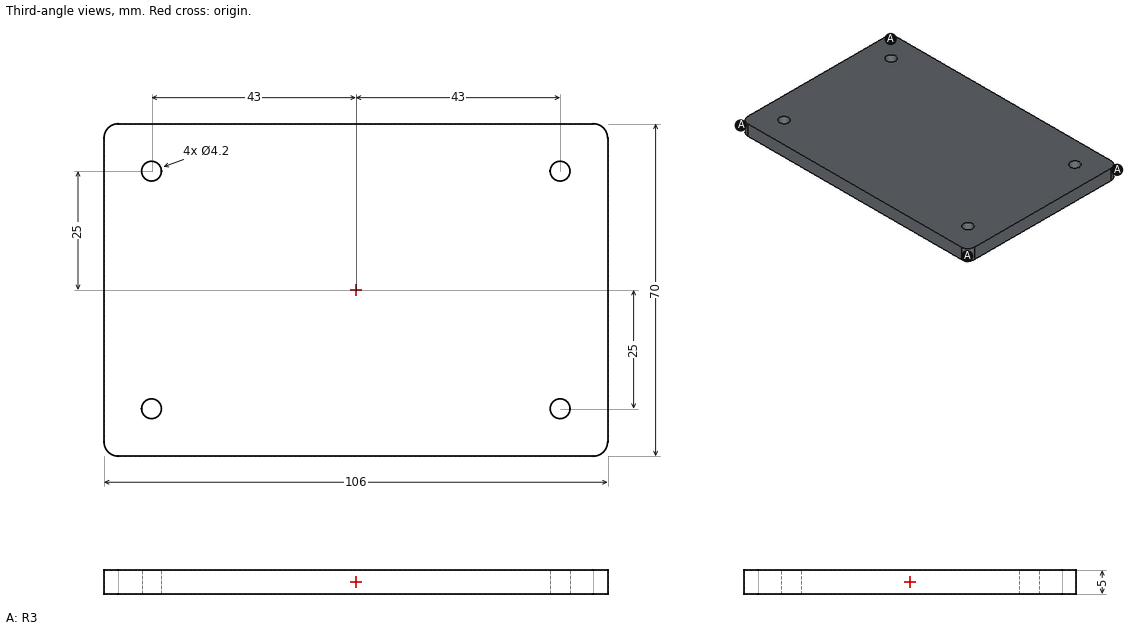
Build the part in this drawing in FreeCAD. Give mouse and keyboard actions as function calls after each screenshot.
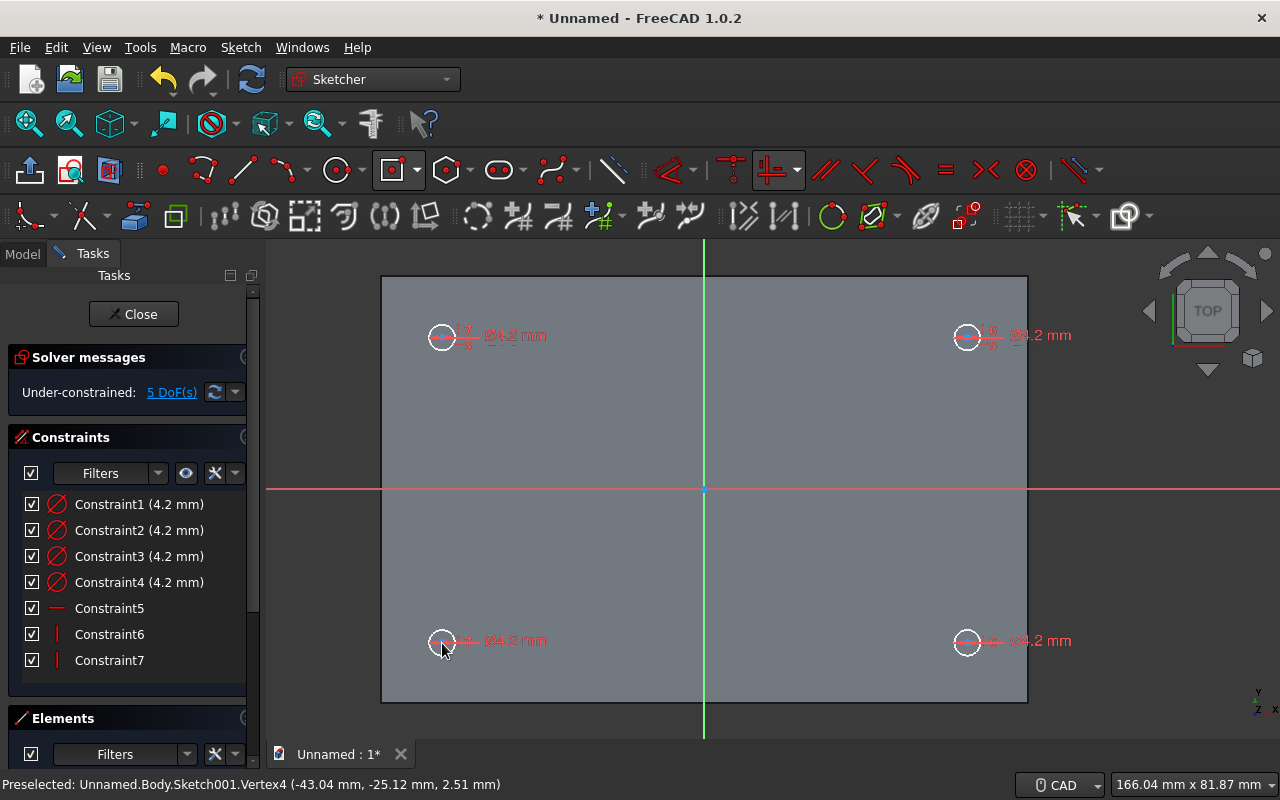
click(967, 643)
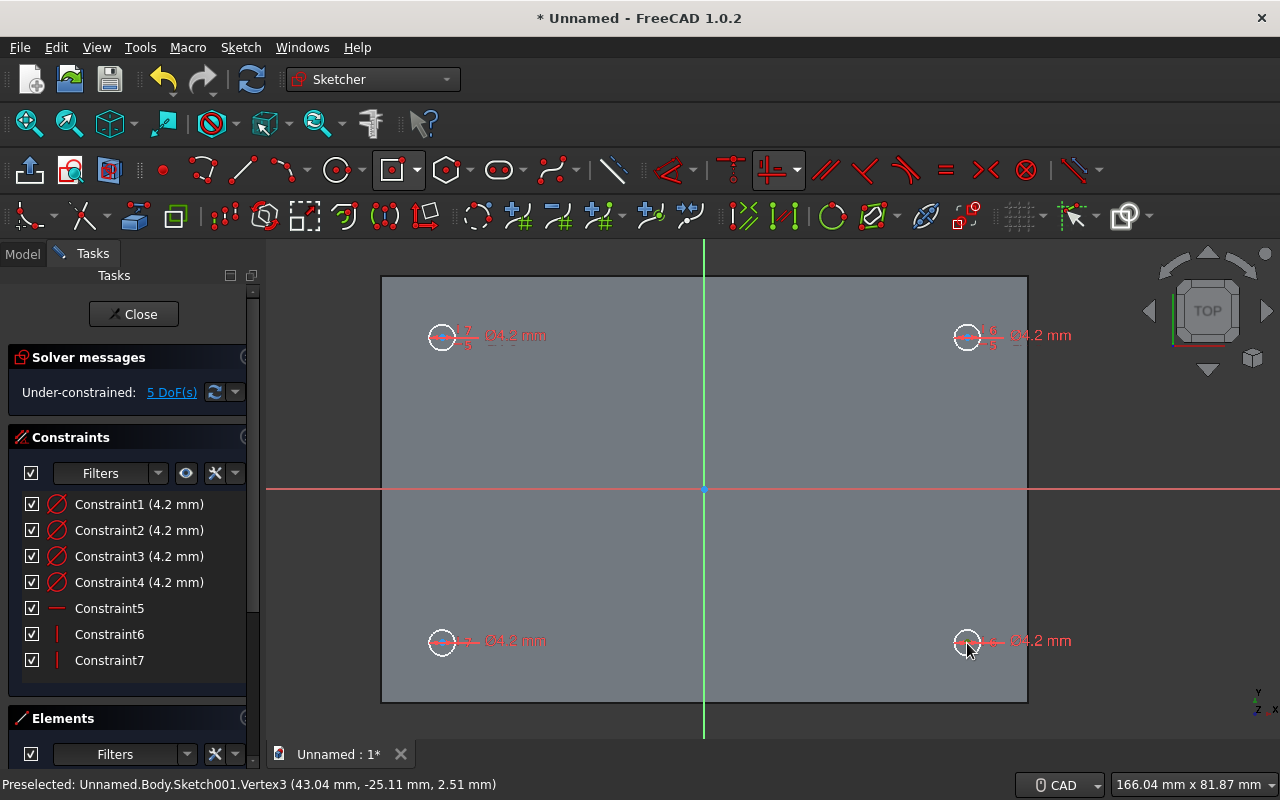
click(442, 643)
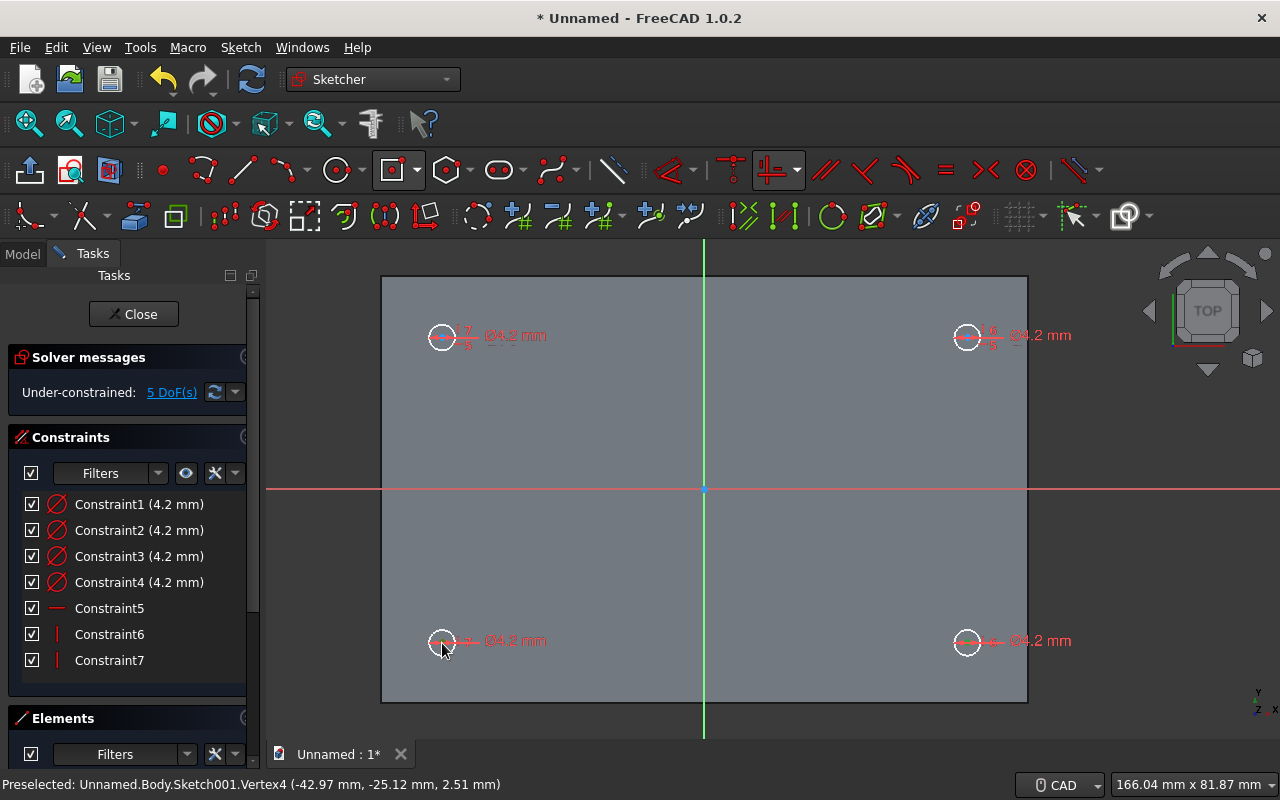
key(h)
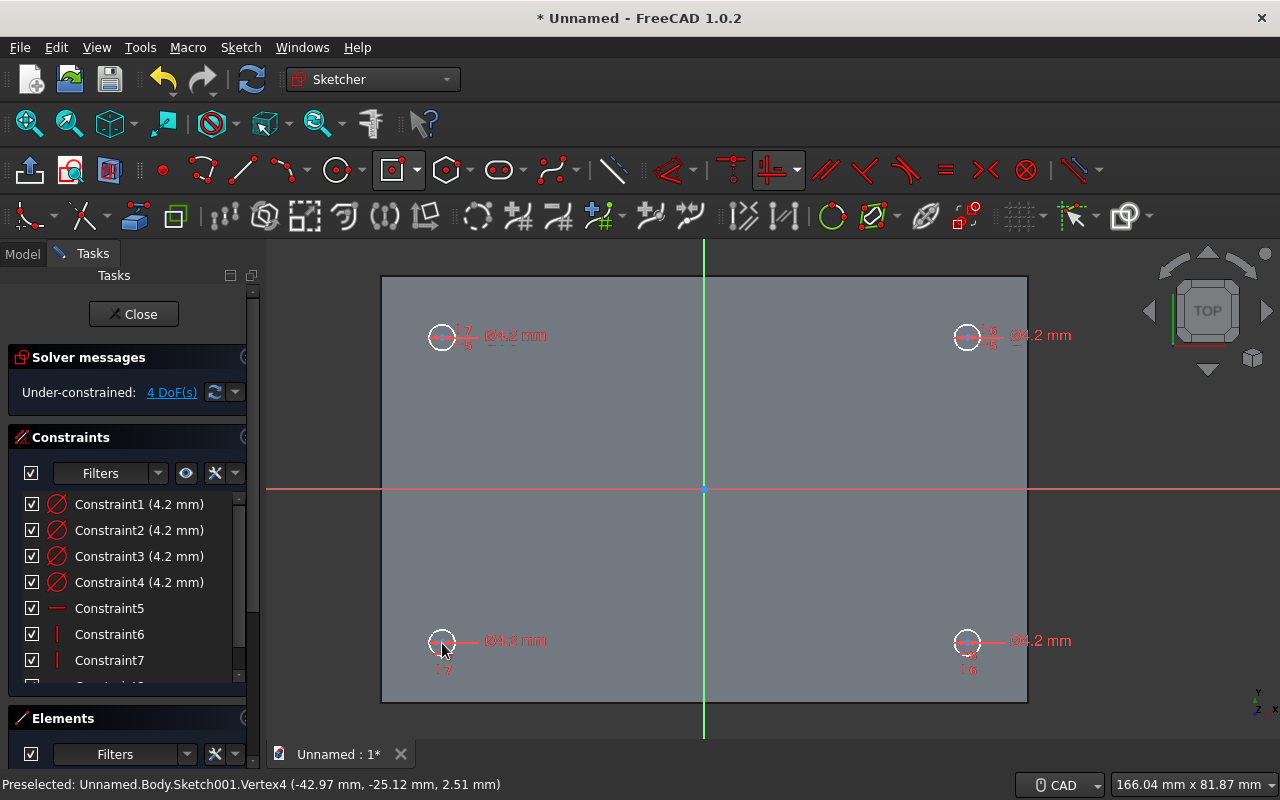
key(d)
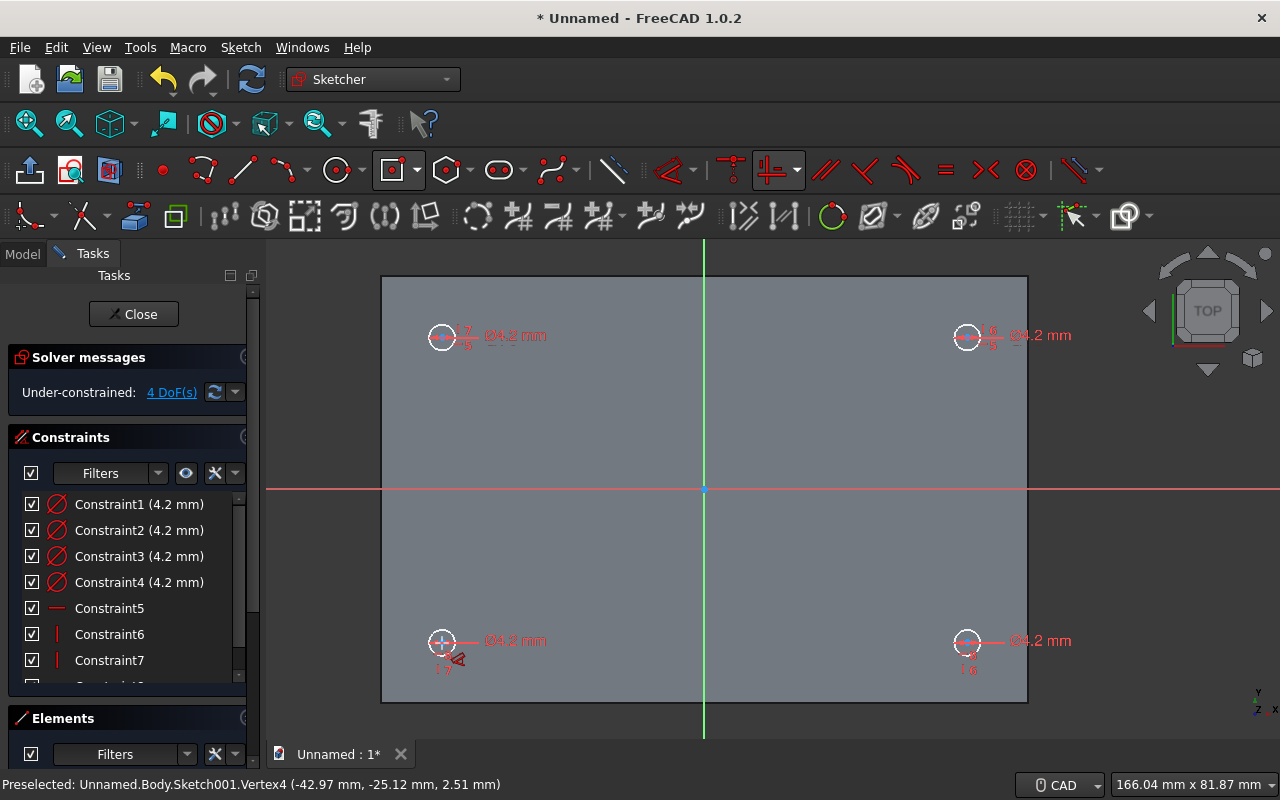
click(442, 338)
click(573, 304)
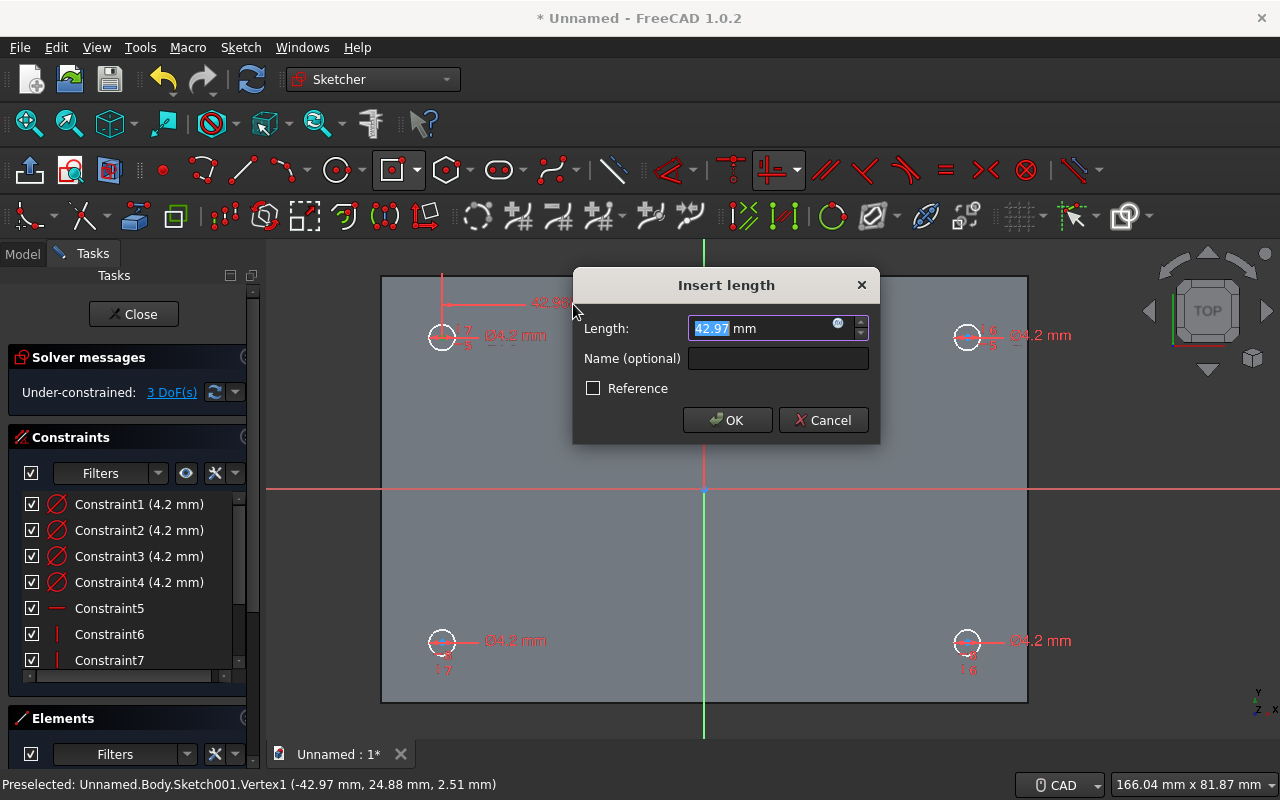
text(43)
key(Return)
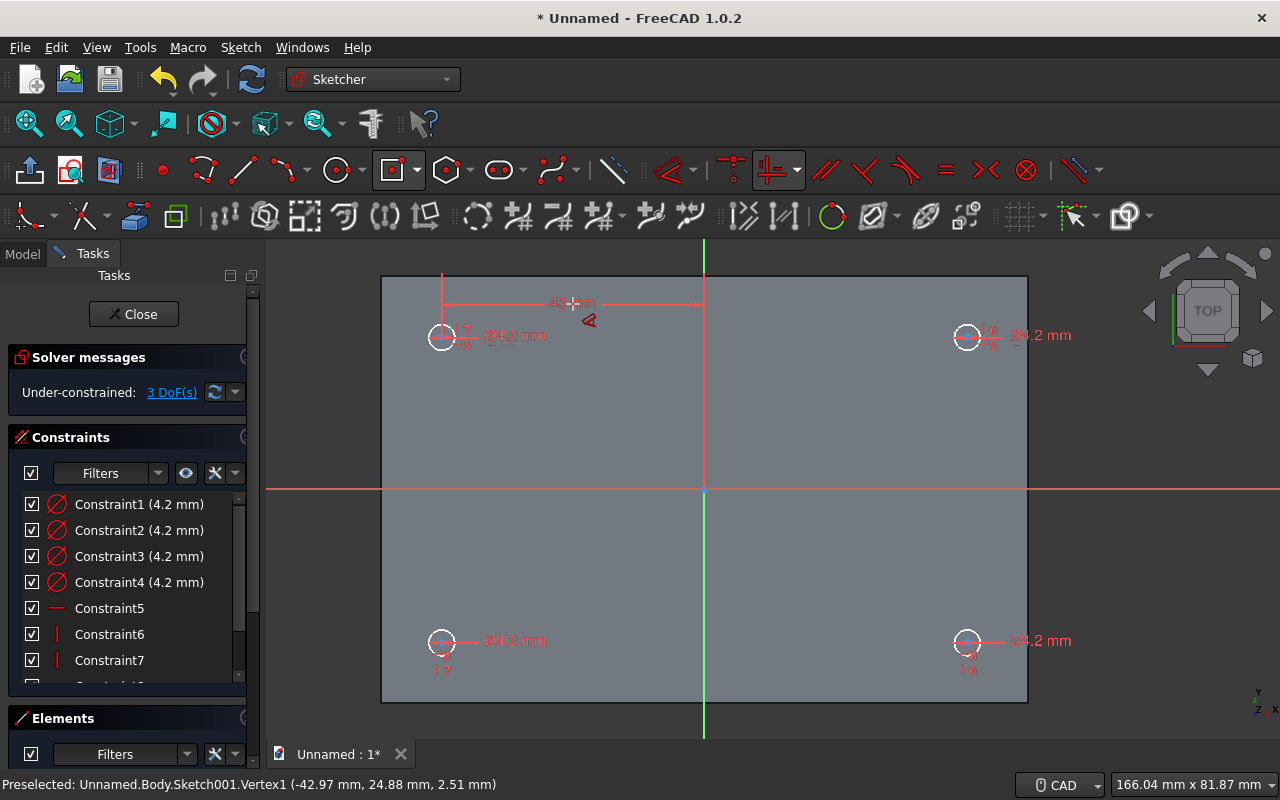
click(442, 338)
click(408, 414)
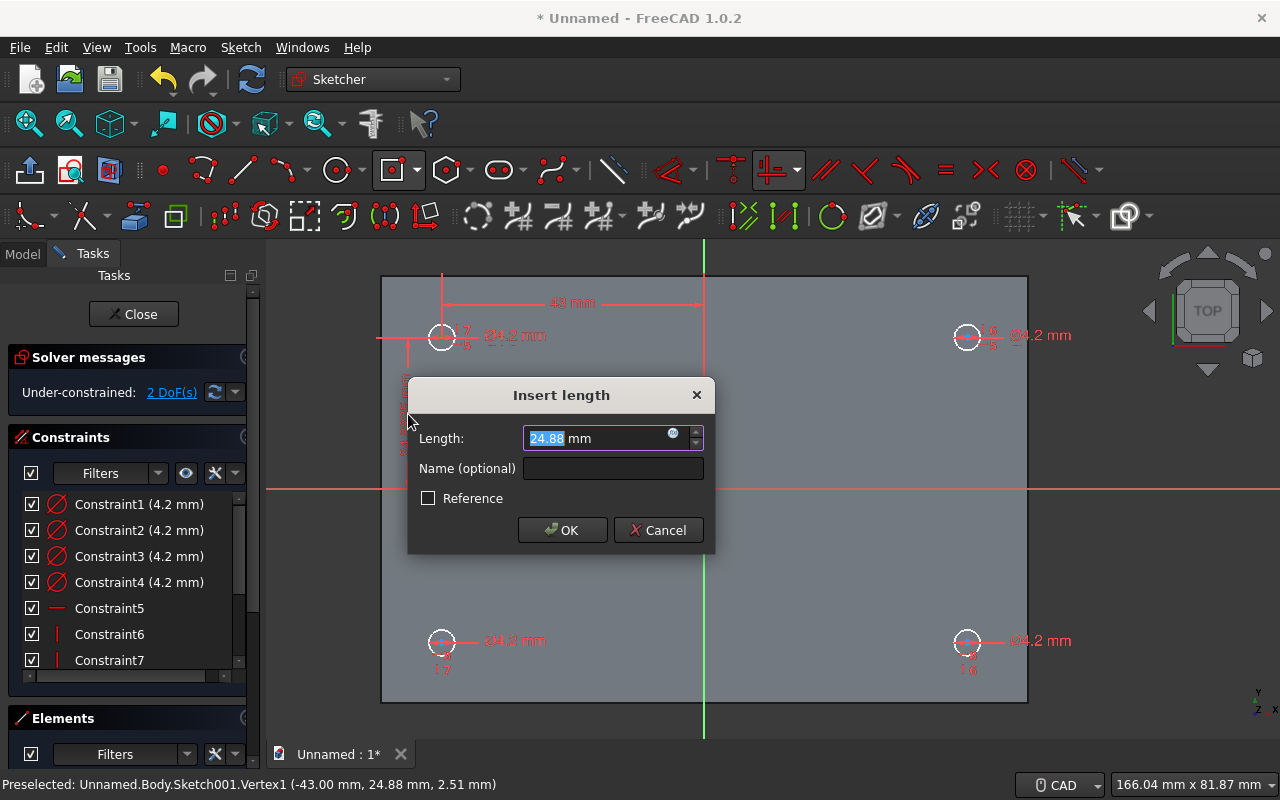
text(25)
key(Return)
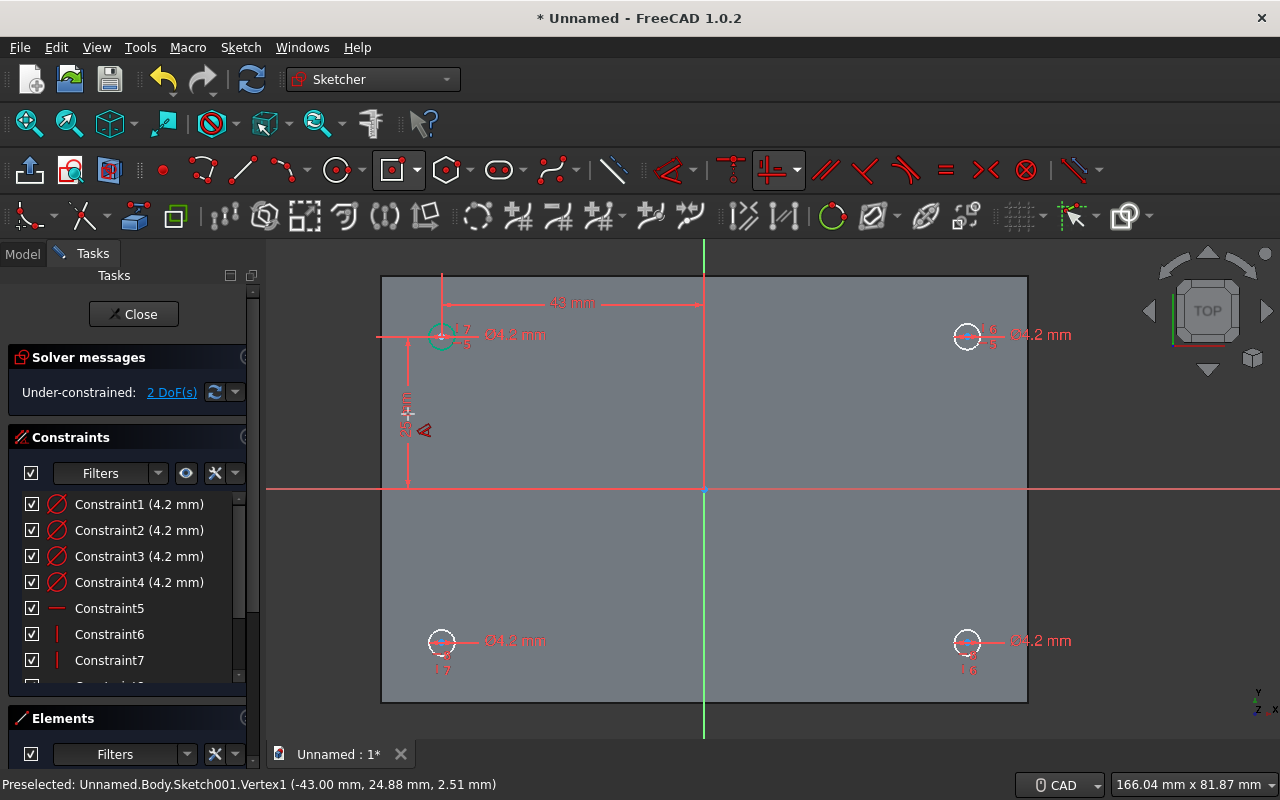
click(967, 337)
click(836, 303)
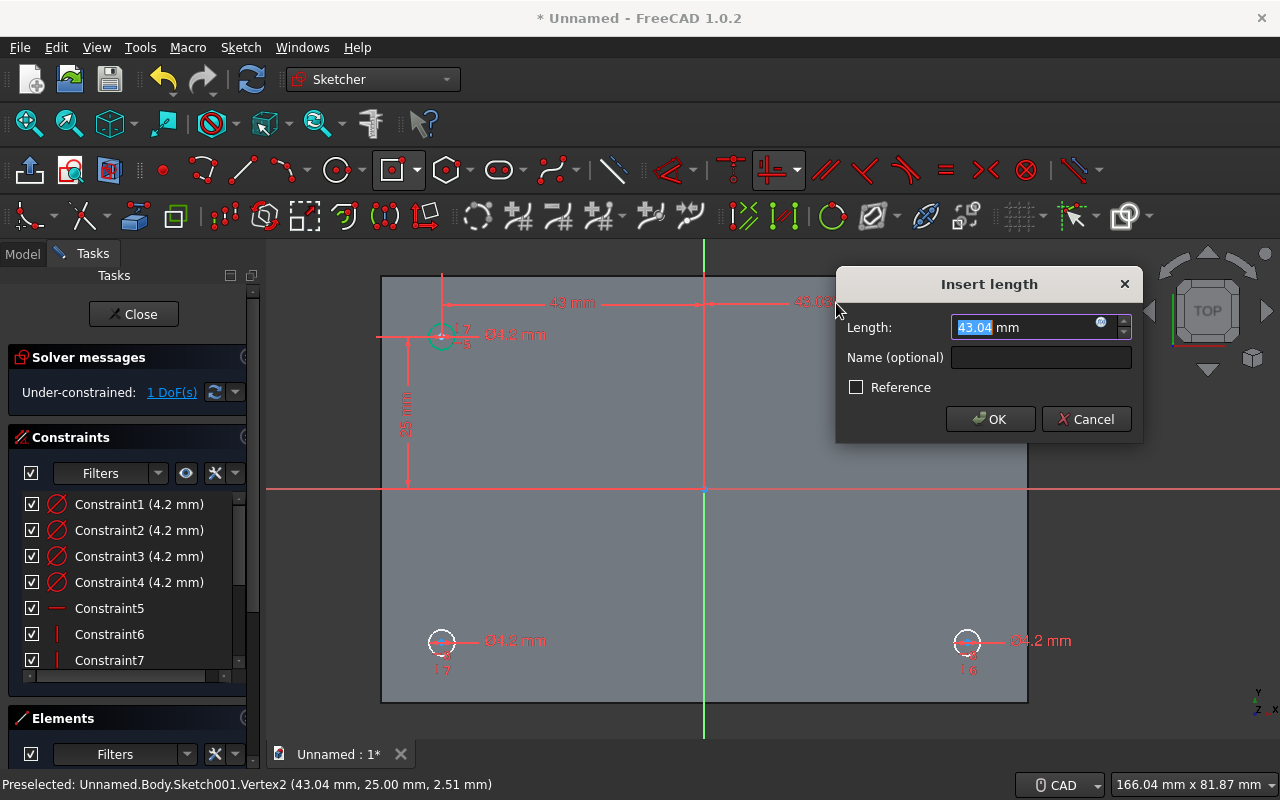
text(43)
key(Return)